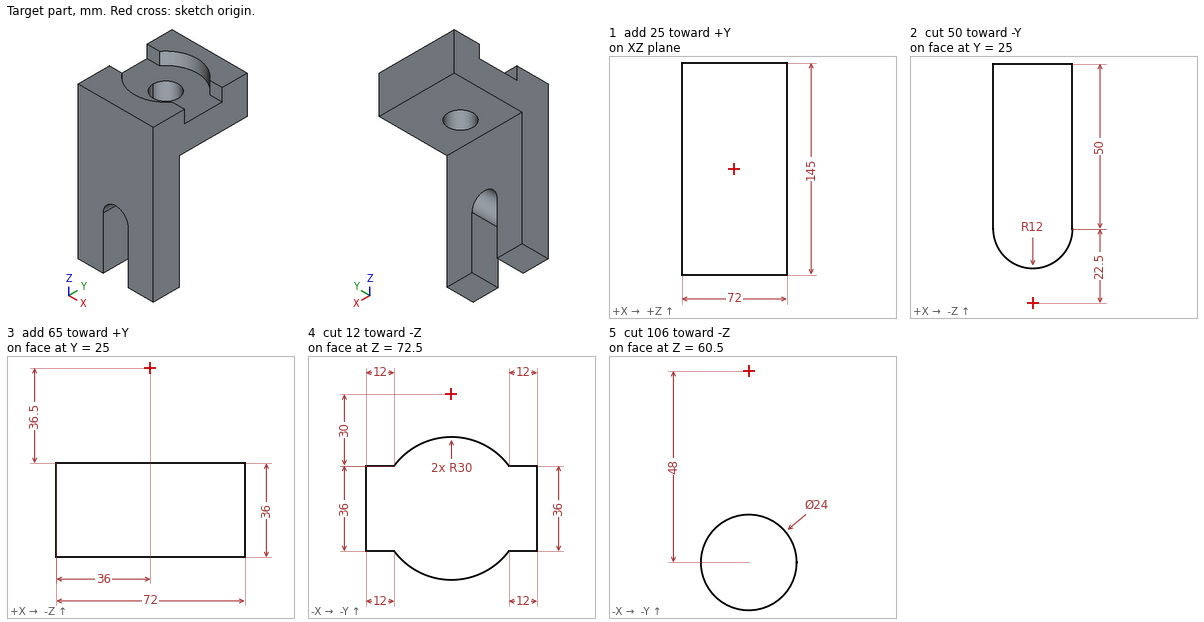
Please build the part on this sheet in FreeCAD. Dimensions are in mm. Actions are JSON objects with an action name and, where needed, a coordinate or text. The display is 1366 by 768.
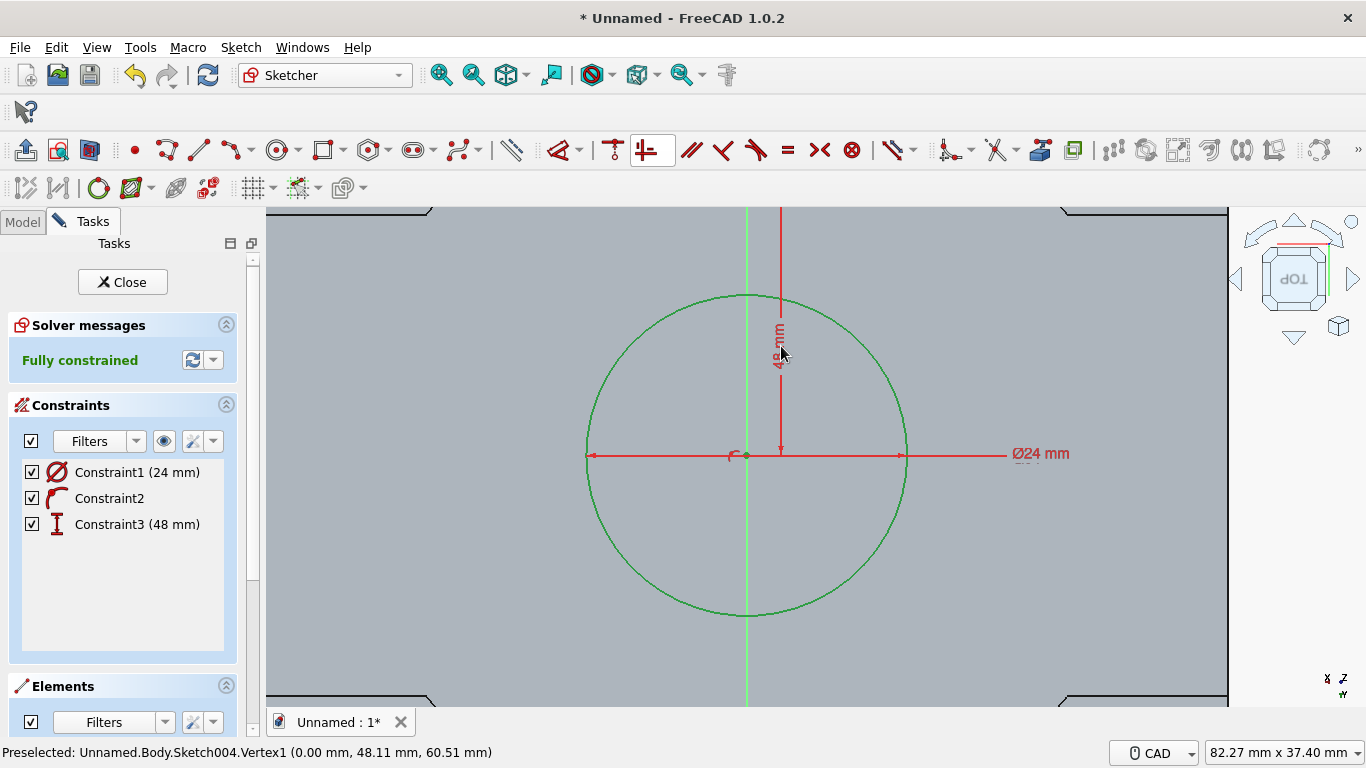
{"action": "left_click", "coordinate": [123, 282]}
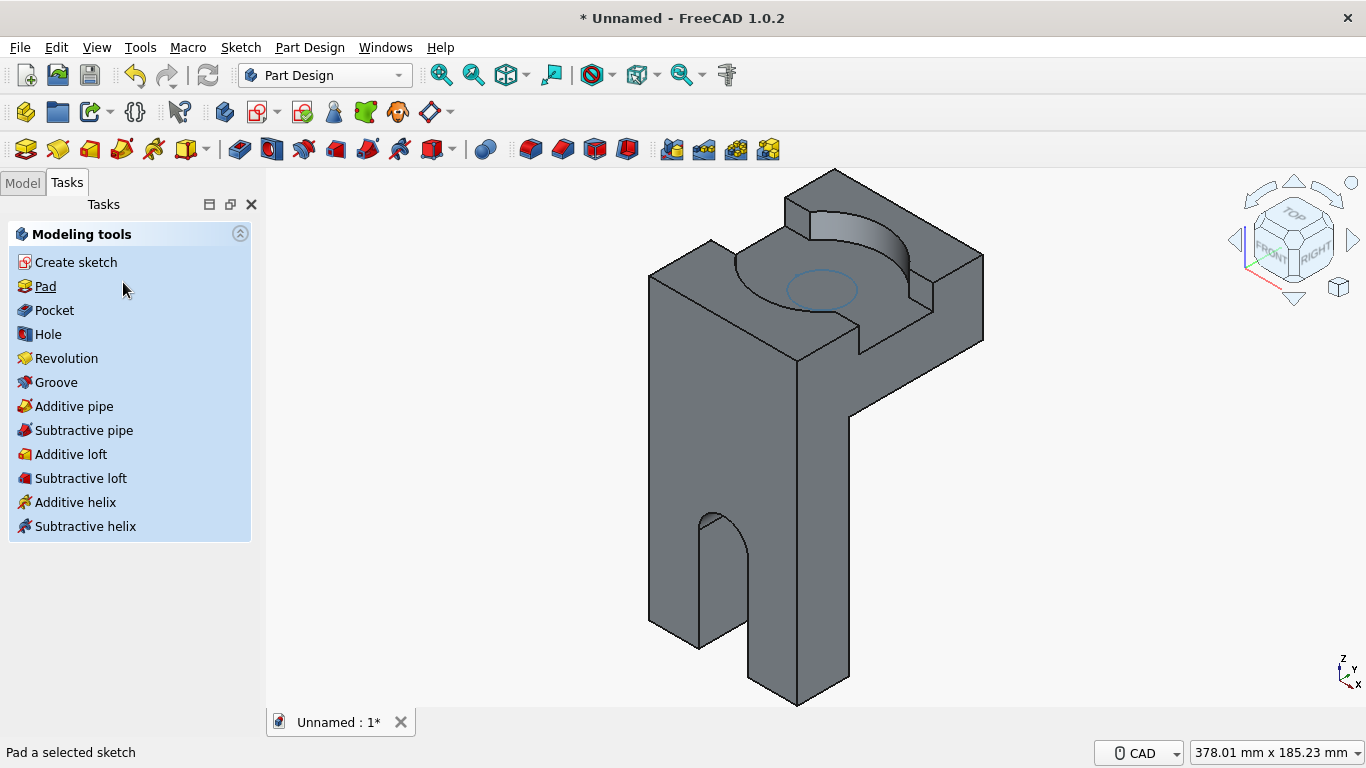
{"action": "left_click", "coordinate": [240, 150]}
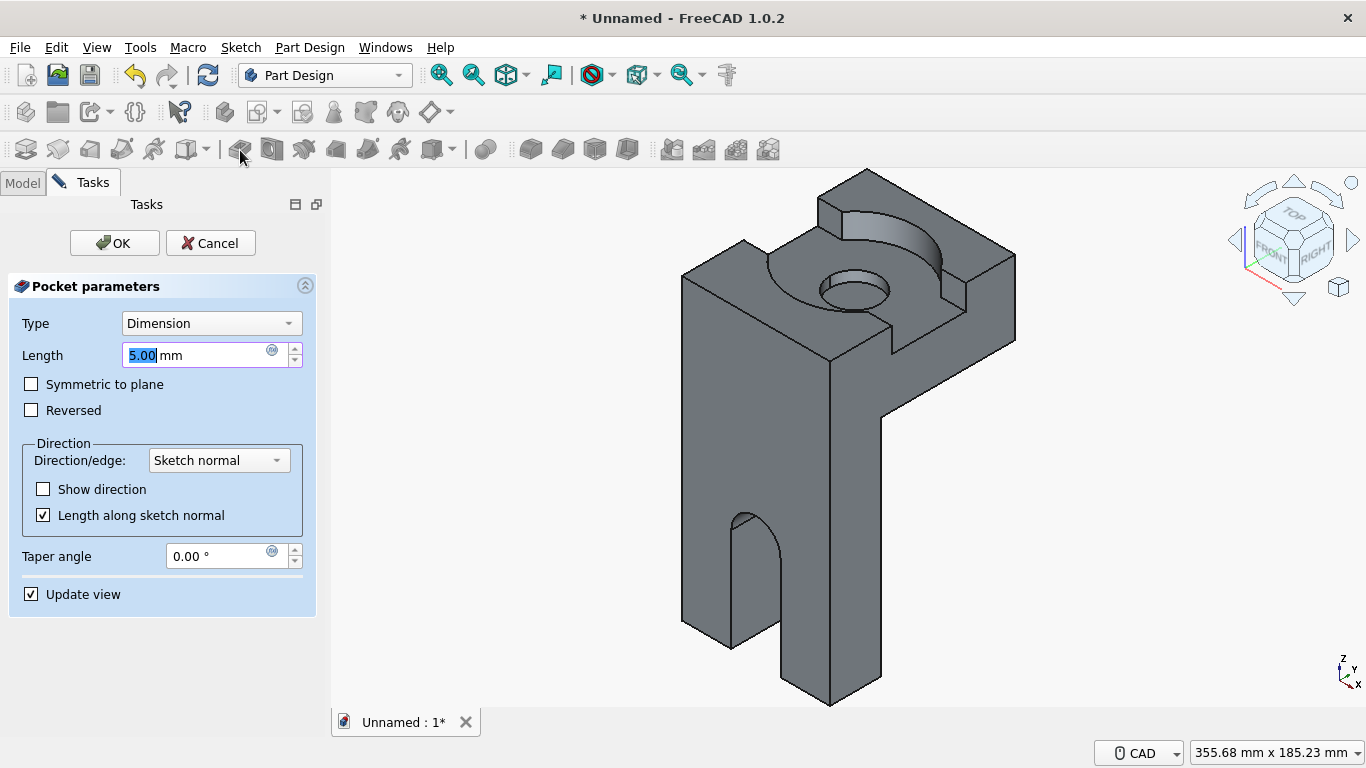
{"action": "type", "text": "106"}
{"action": "key", "text": "Tab"}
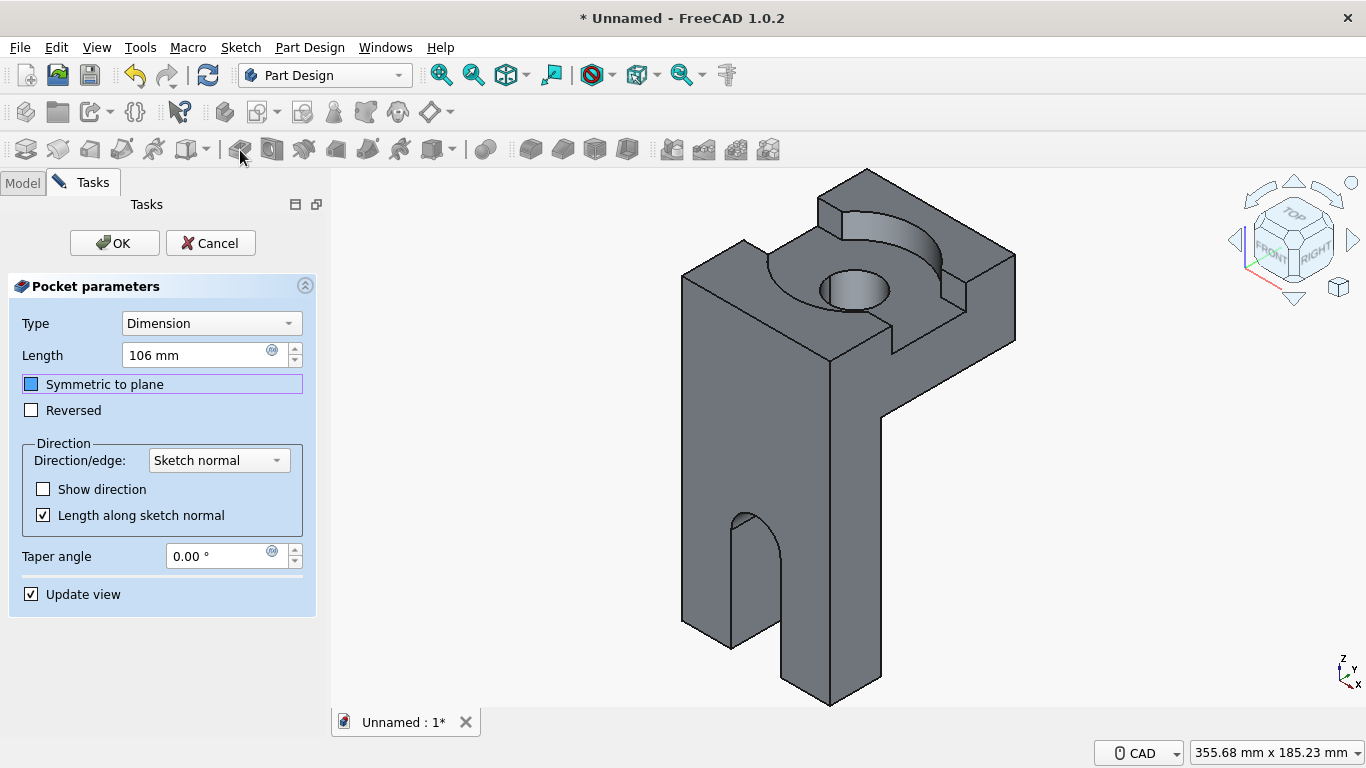
{"action": "left_click", "coordinate": [115, 243]}